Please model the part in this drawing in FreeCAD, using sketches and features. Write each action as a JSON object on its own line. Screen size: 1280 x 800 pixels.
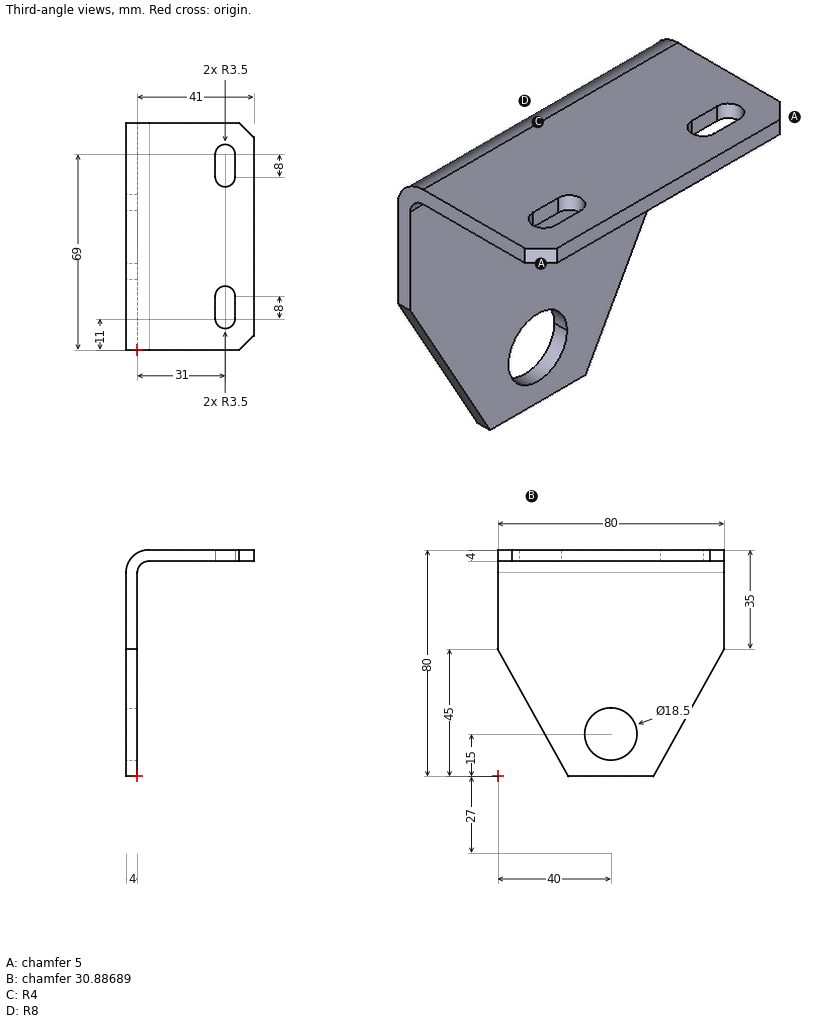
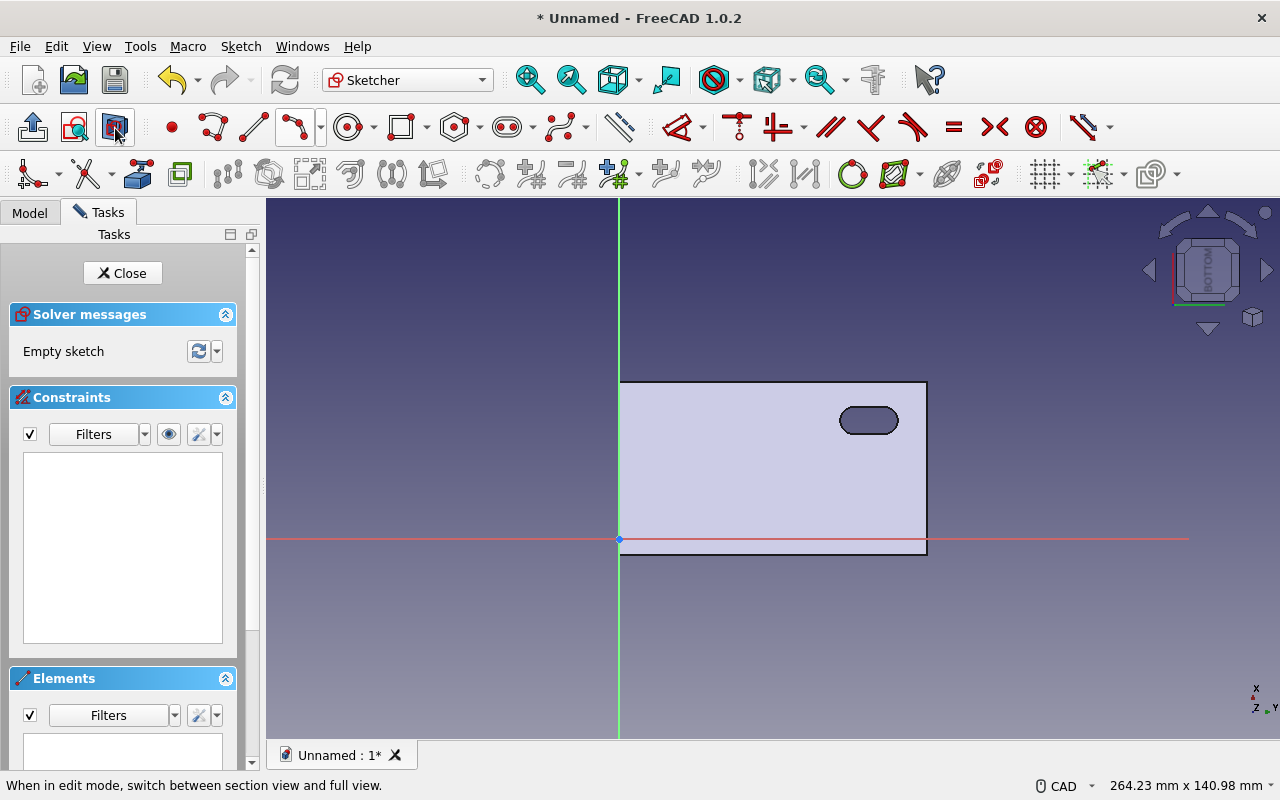
{"action": "scroll", "coordinate": [638, 476], "scroll_direction": "up", "scroll_amount": 5}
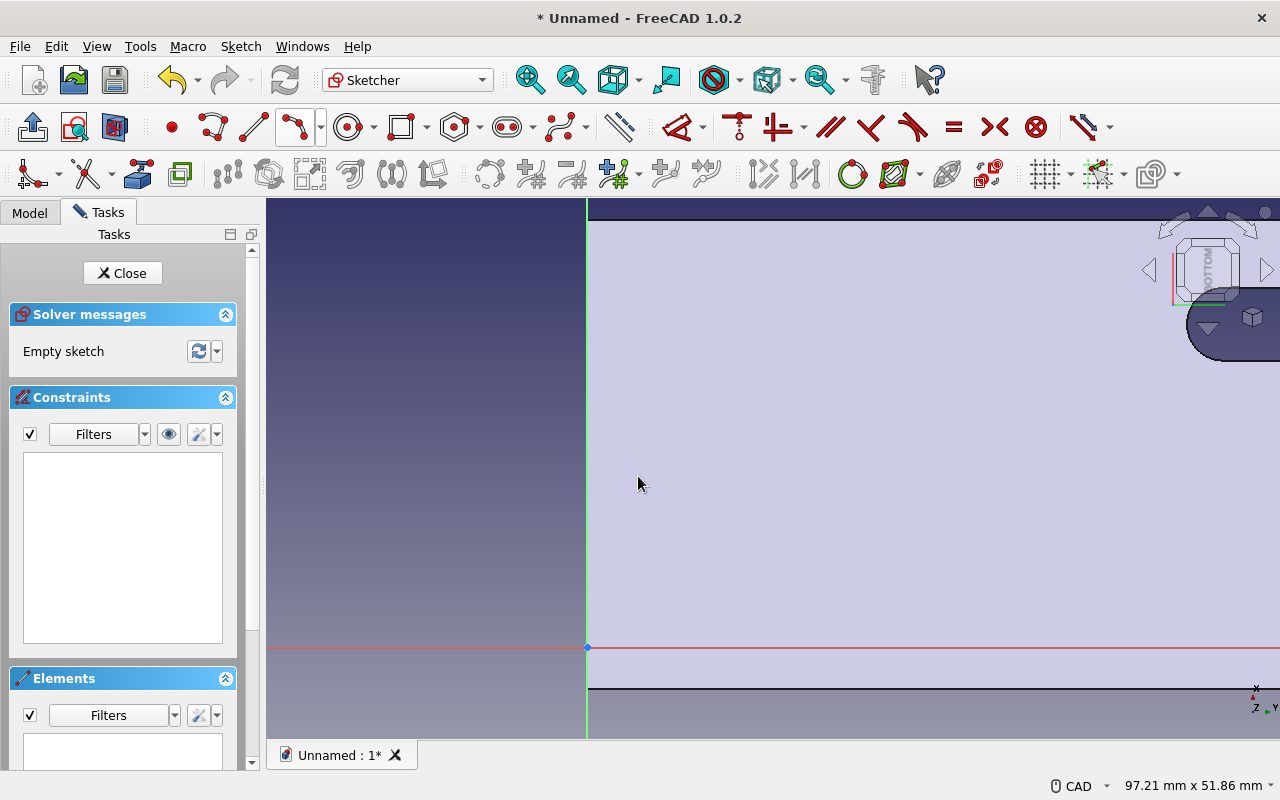
{"action": "left_click", "coordinate": [506, 128]}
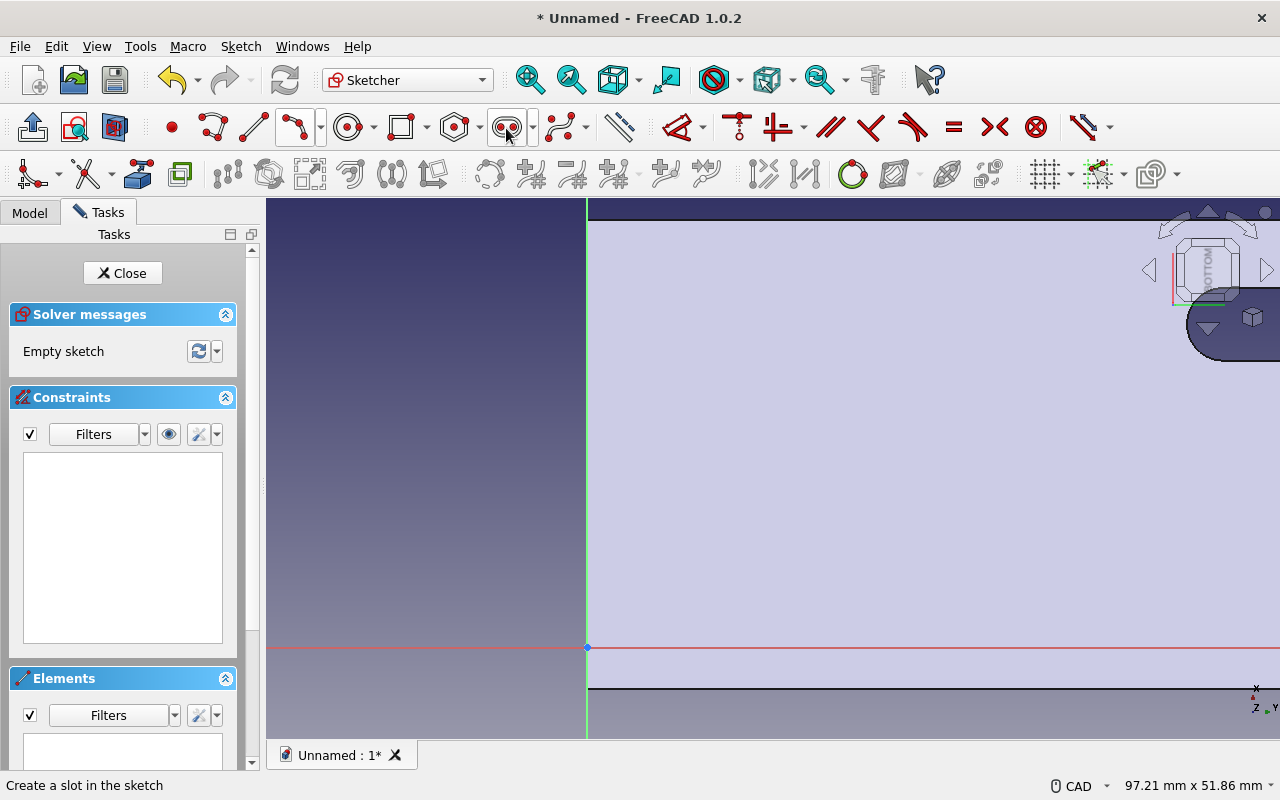
{"action": "left_click", "coordinate": [702, 324]}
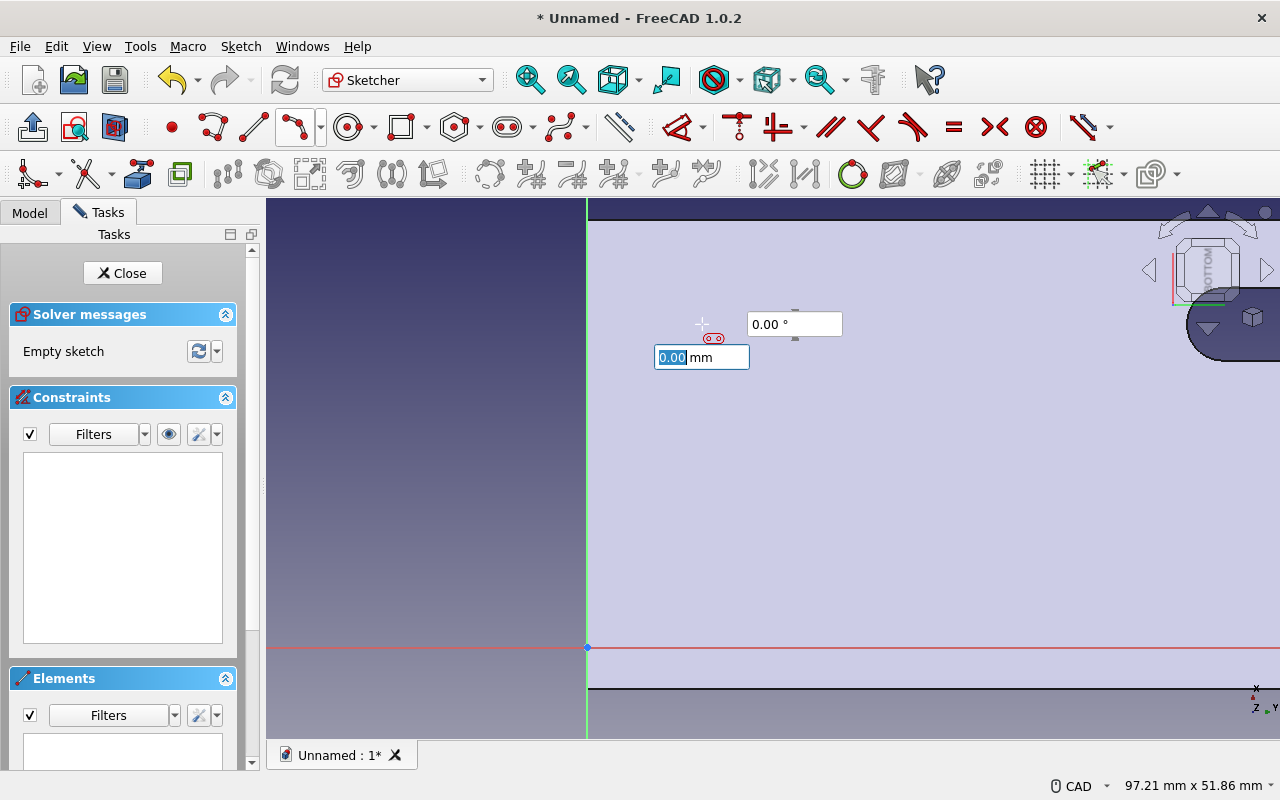
{"action": "left_click", "coordinate": [785, 324]}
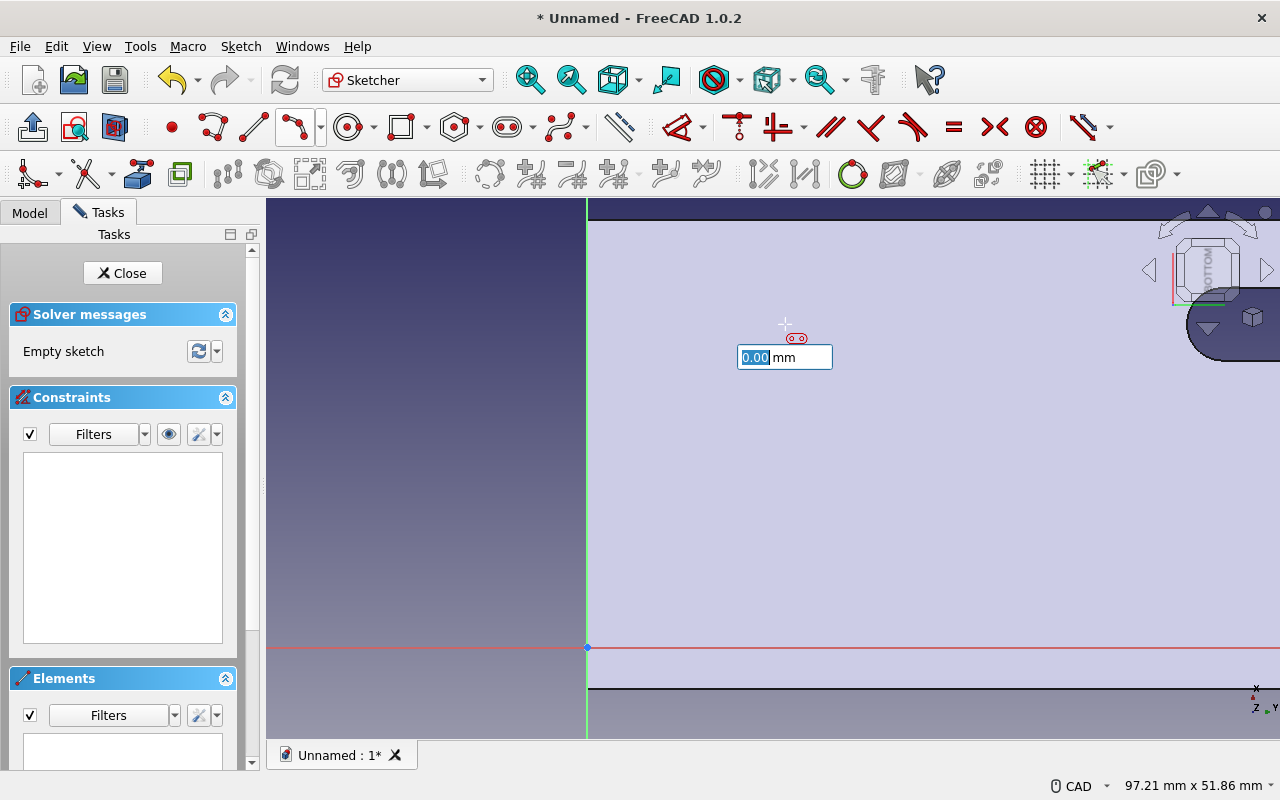
{"action": "left_click", "coordinate": [744, 288]}
{"action": "key", "text": "Escape"}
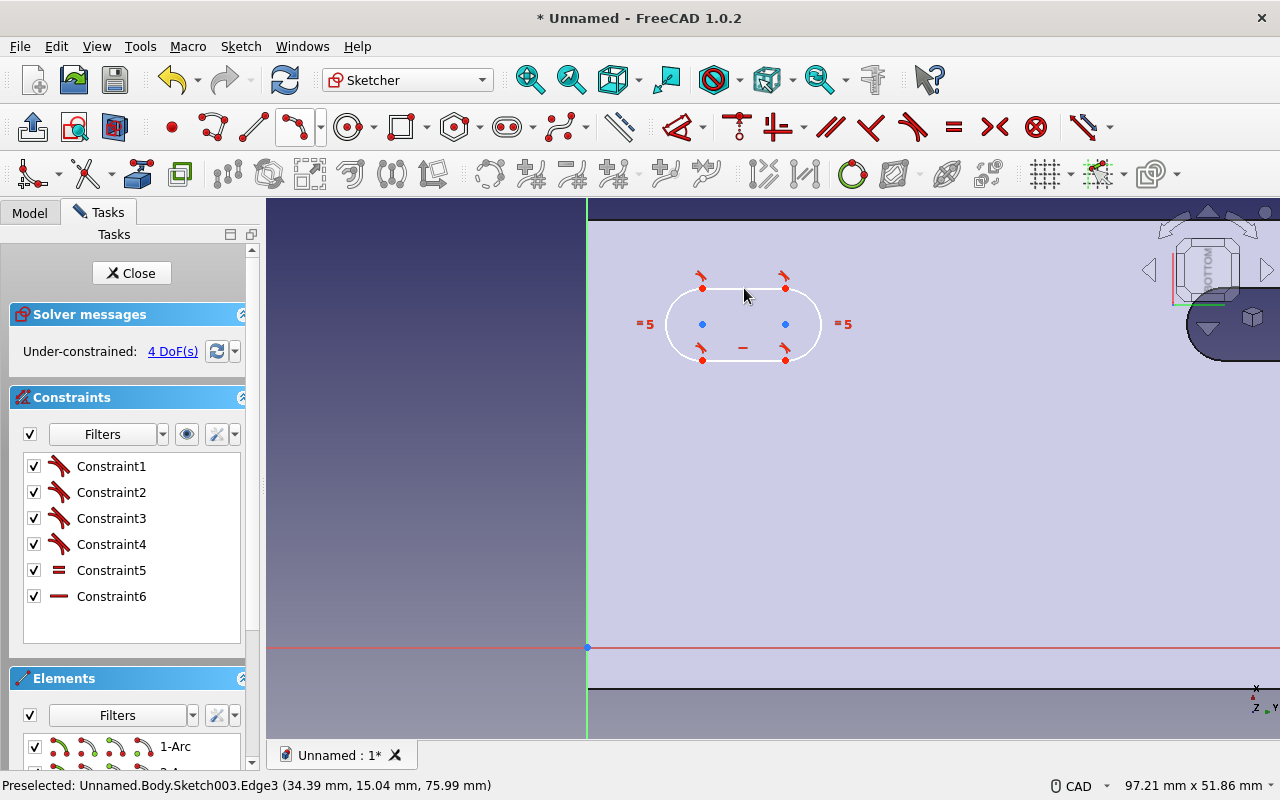
{"action": "key", "text": "d"}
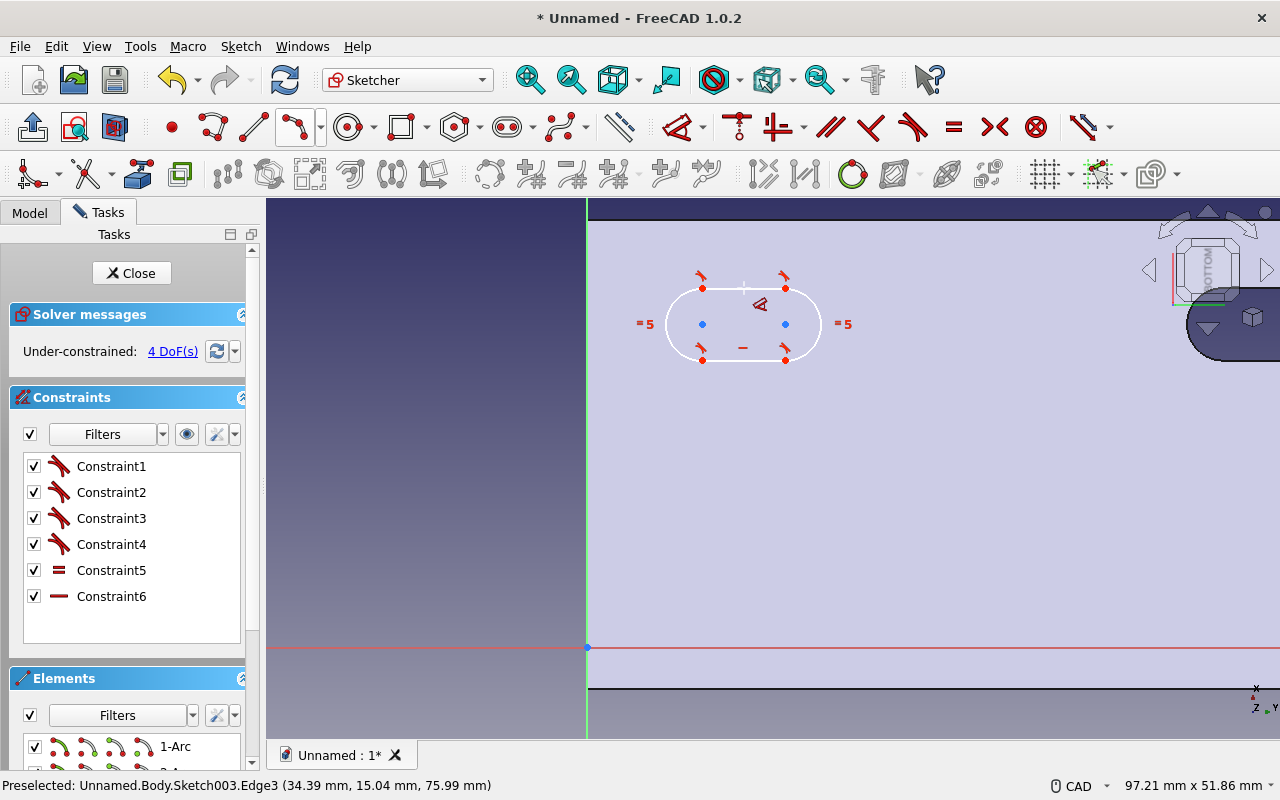
{"action": "left_click", "coordinate": [673, 304]}
{"action": "left_click", "coordinate": [647, 285]}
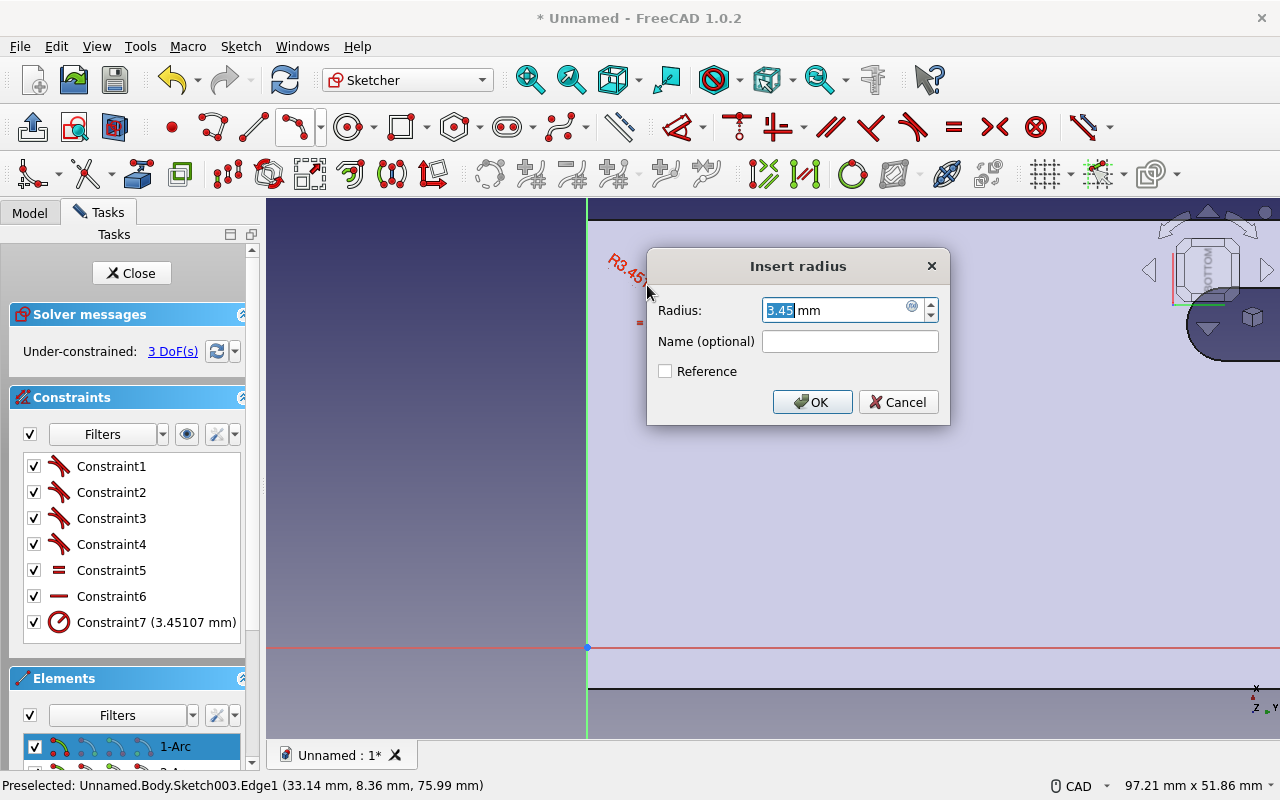
{"action": "type", "text": "3.5"}
{"action": "key", "text": "Return"}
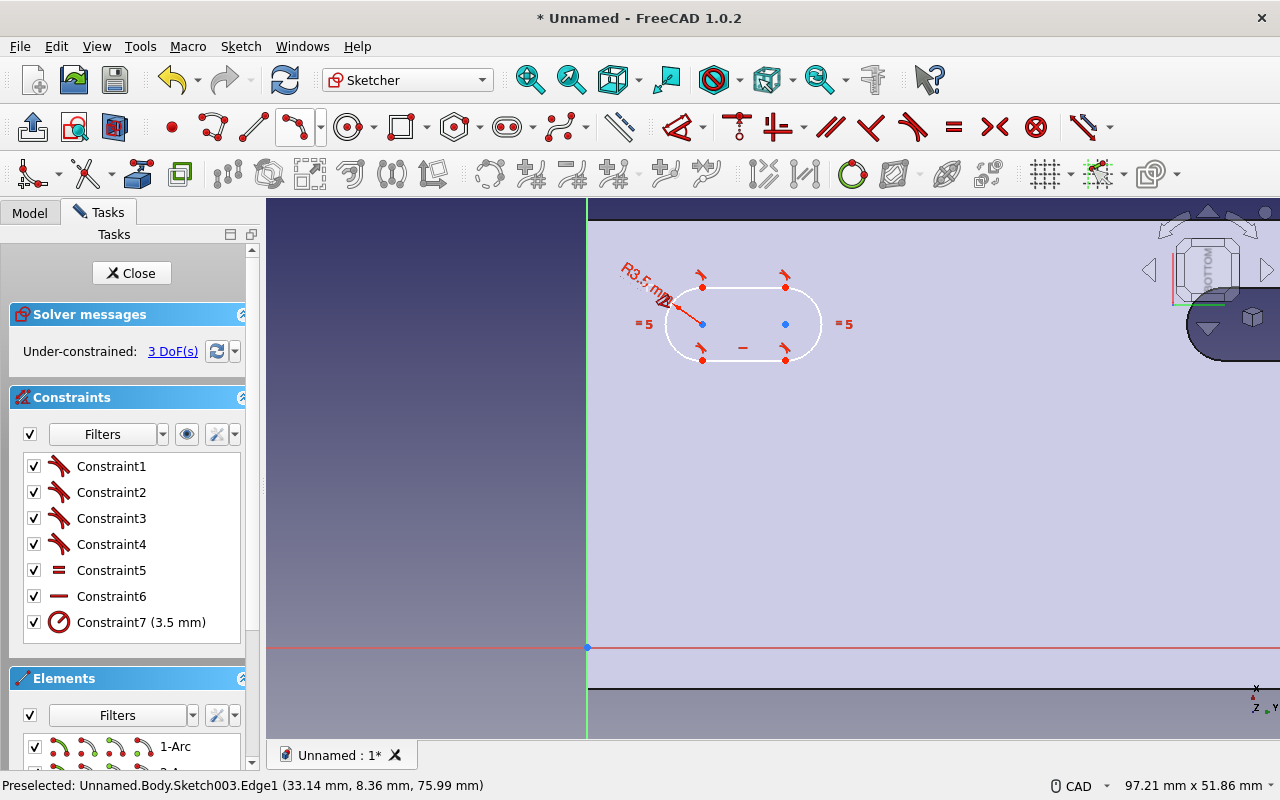
{"action": "left_click", "coordinate": [727, 288]}
{"action": "left_click", "coordinate": [743, 254]}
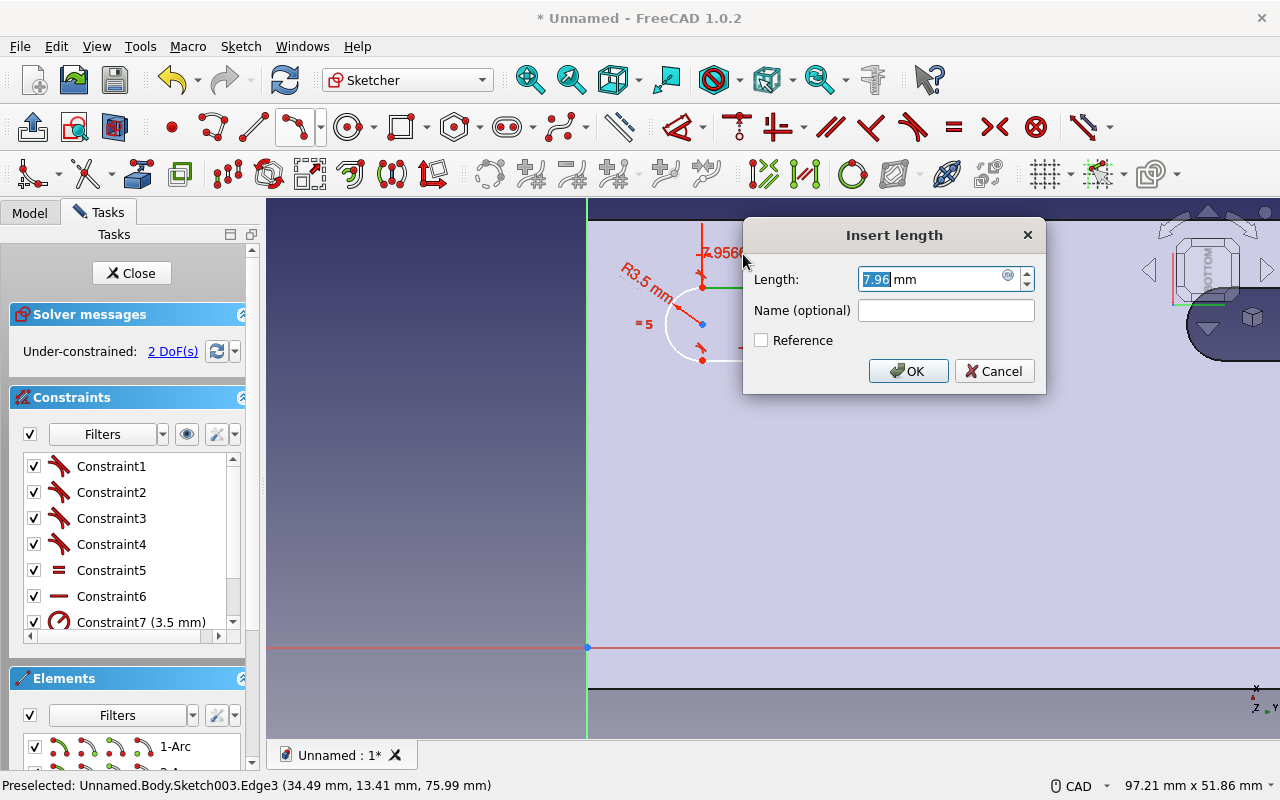
{"action": "type", "text": "8"}
{"action": "key", "text": "Return"}